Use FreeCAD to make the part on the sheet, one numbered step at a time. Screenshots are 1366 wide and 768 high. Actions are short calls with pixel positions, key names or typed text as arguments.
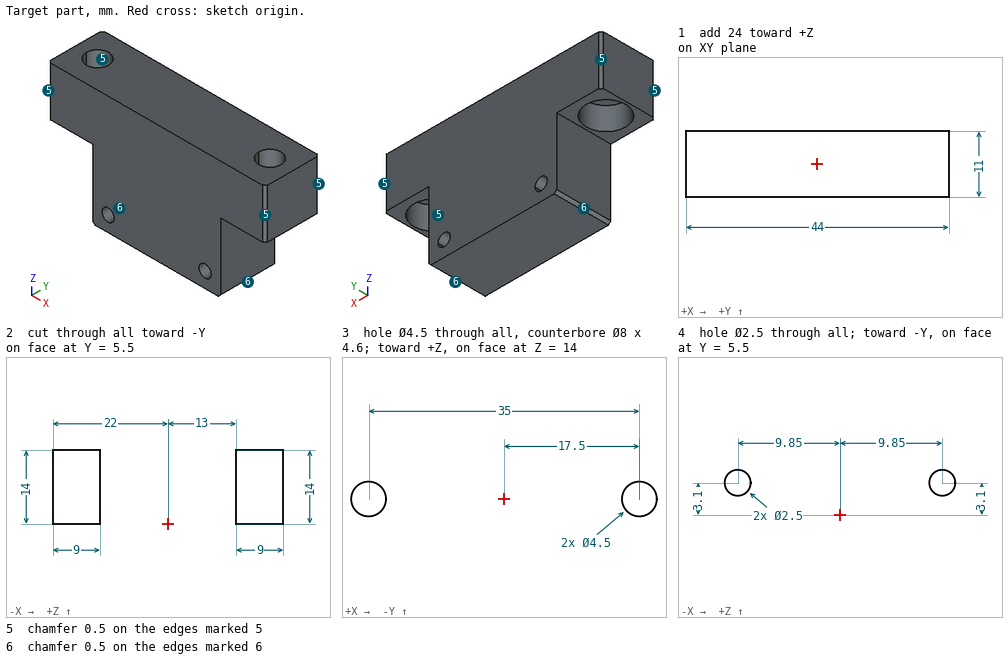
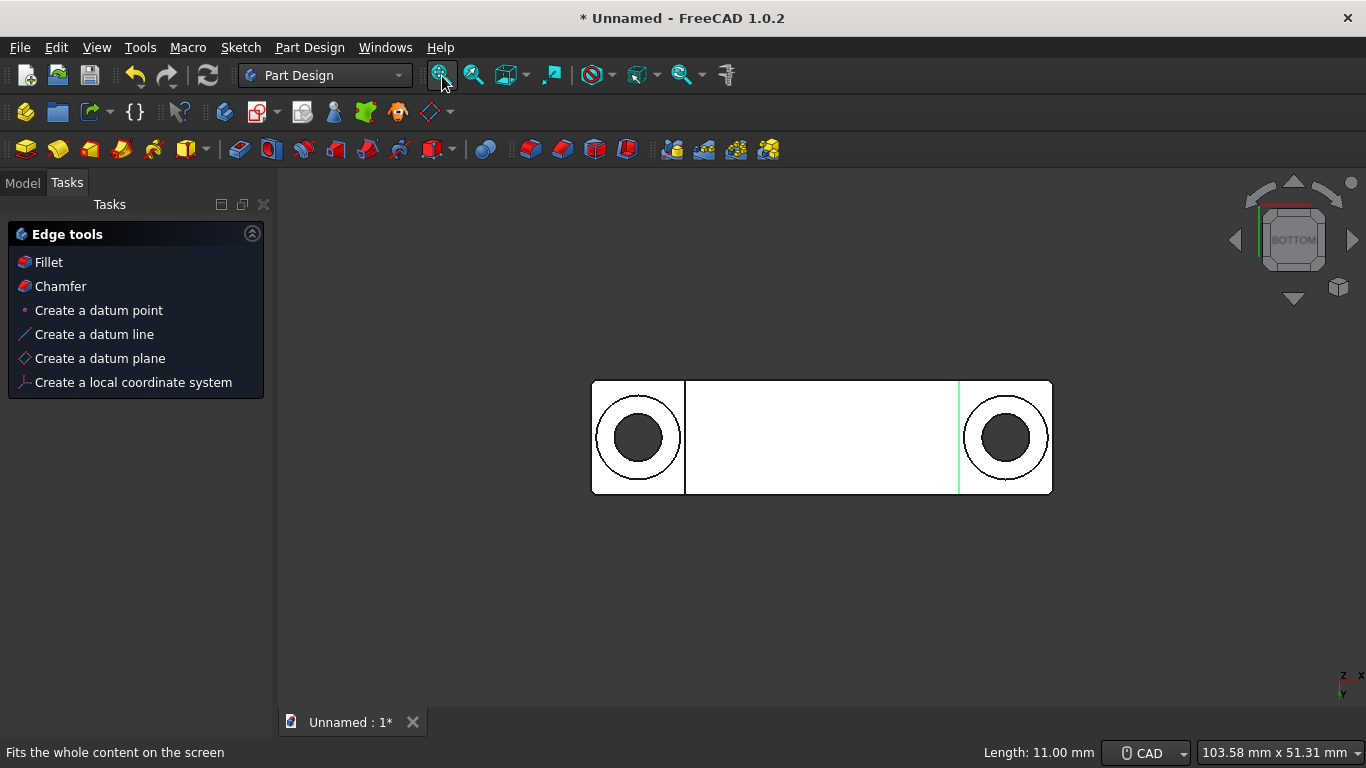
click(442, 76)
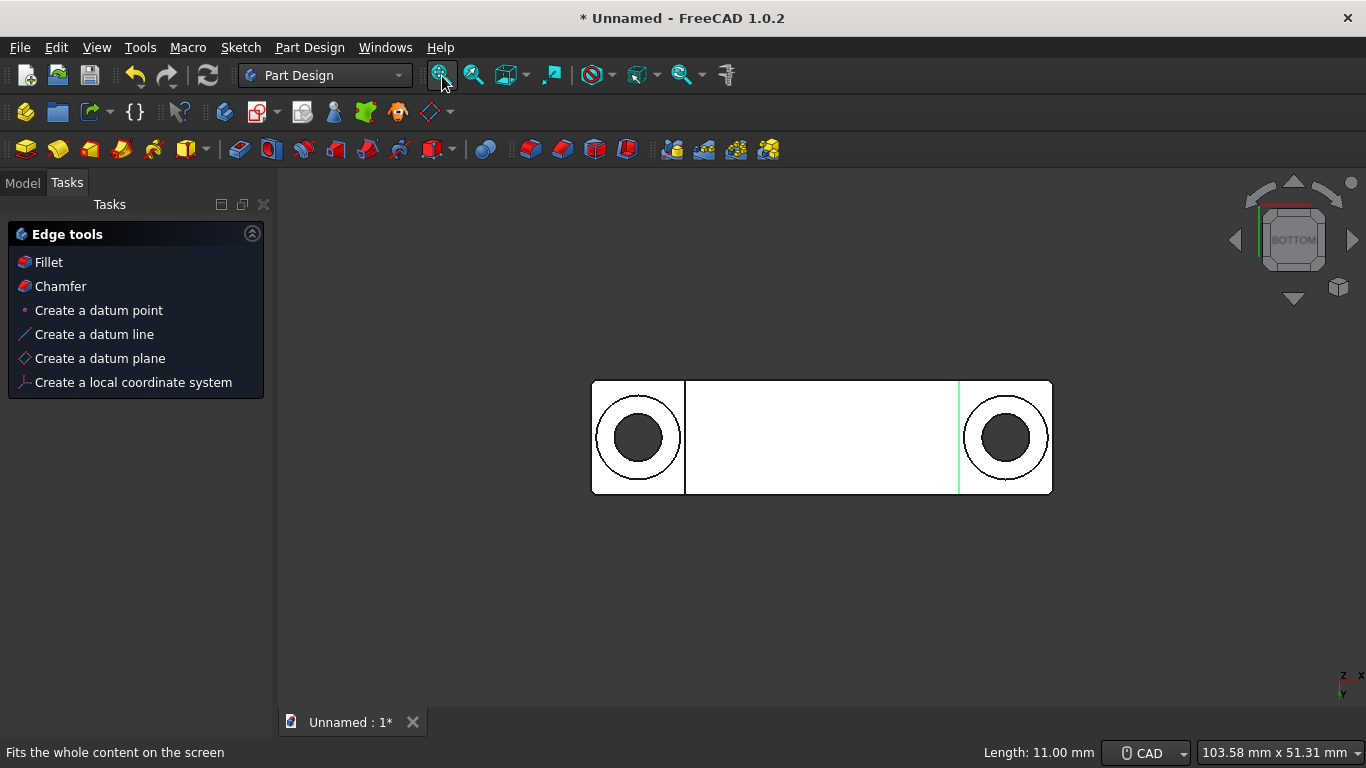
click(685, 436, ctrl)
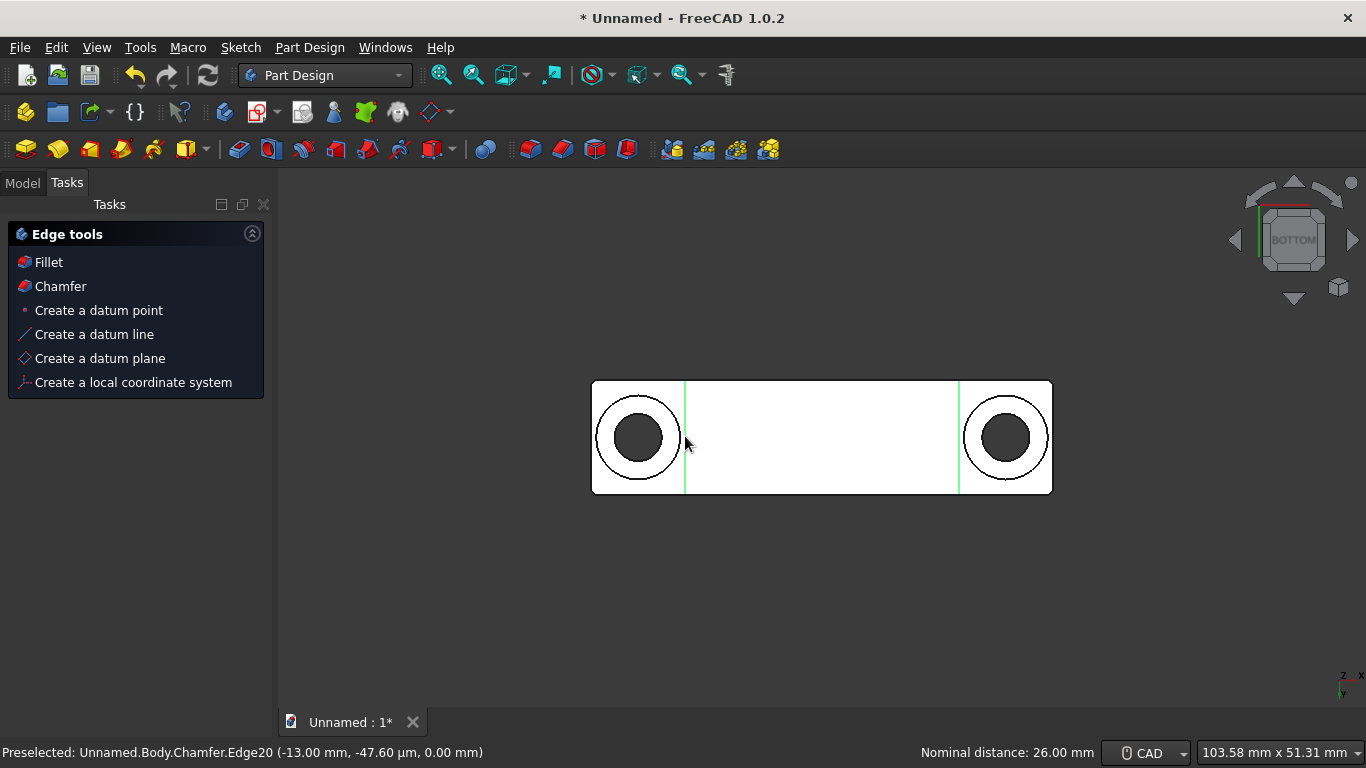
click(564, 150)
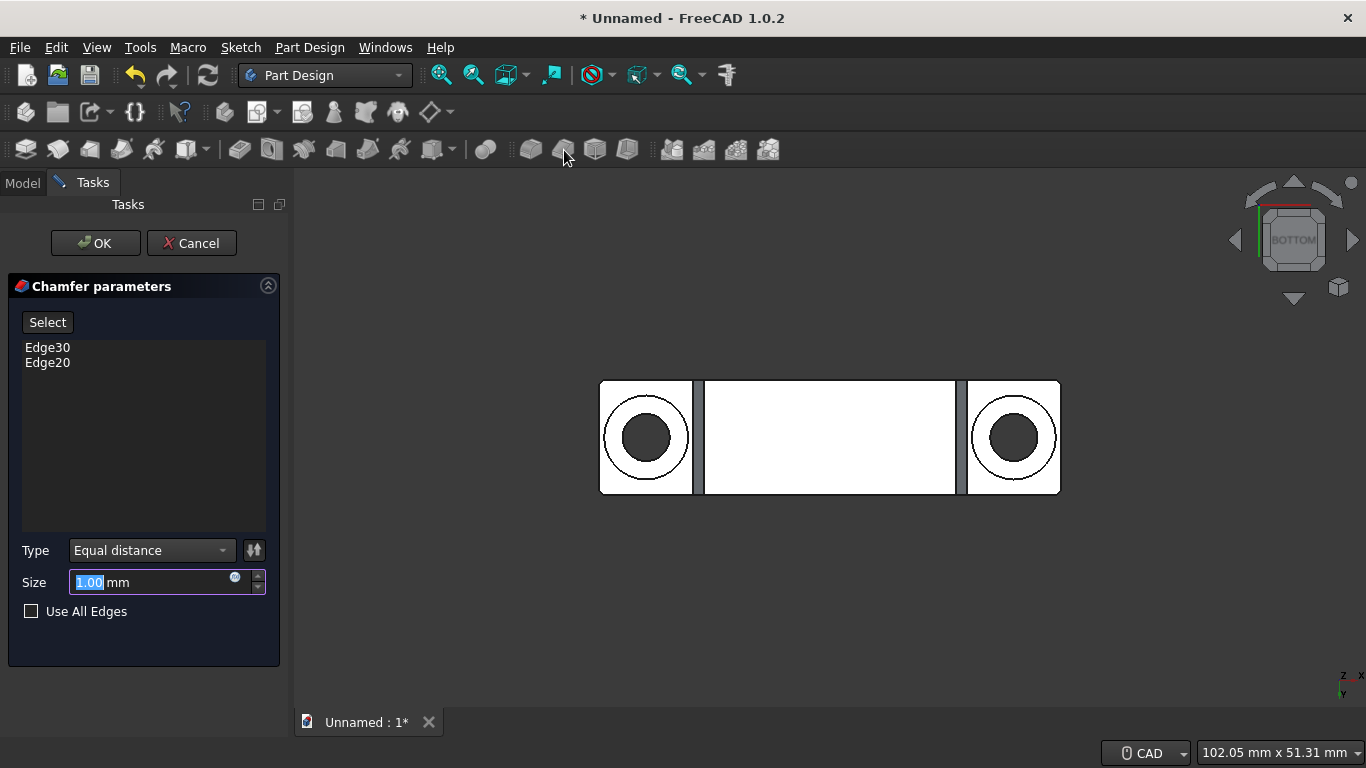
text(0.5)
key(Tab)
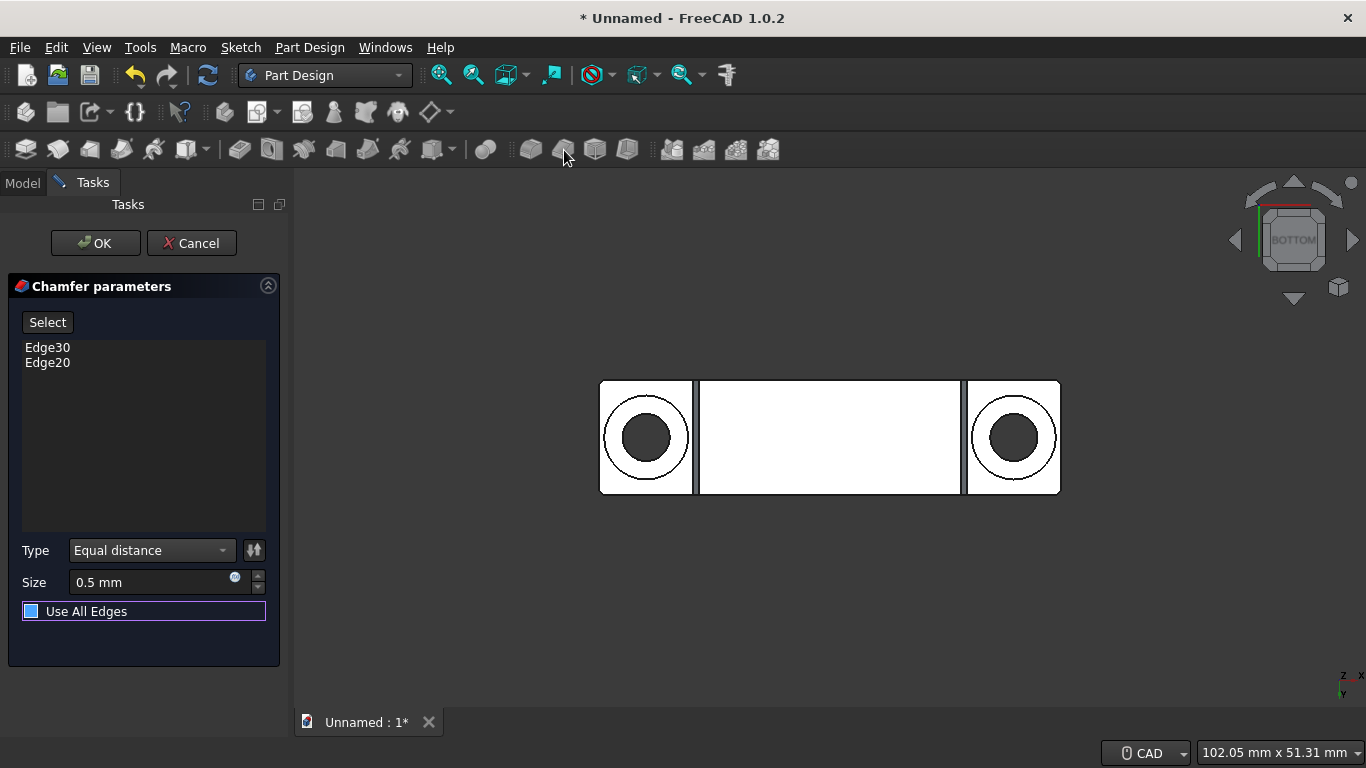
click(96, 243)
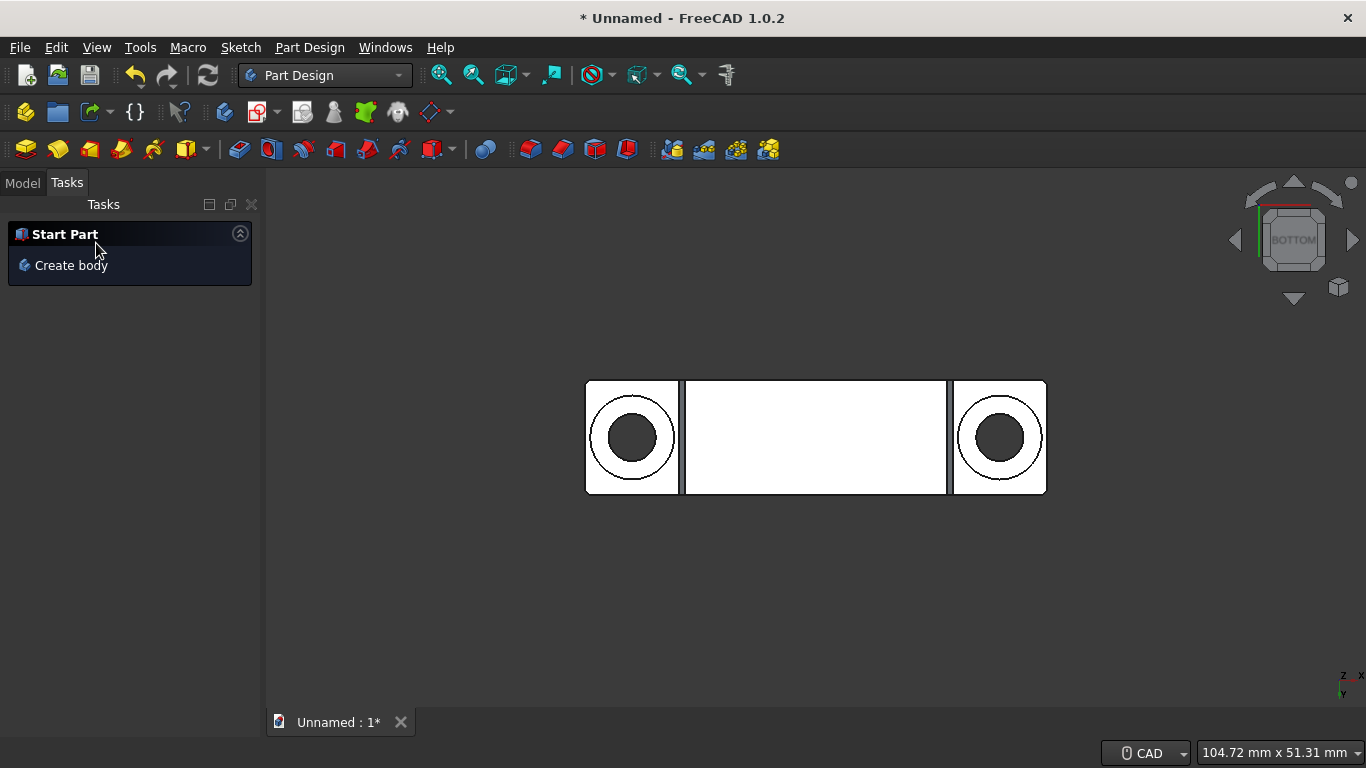
key(0)